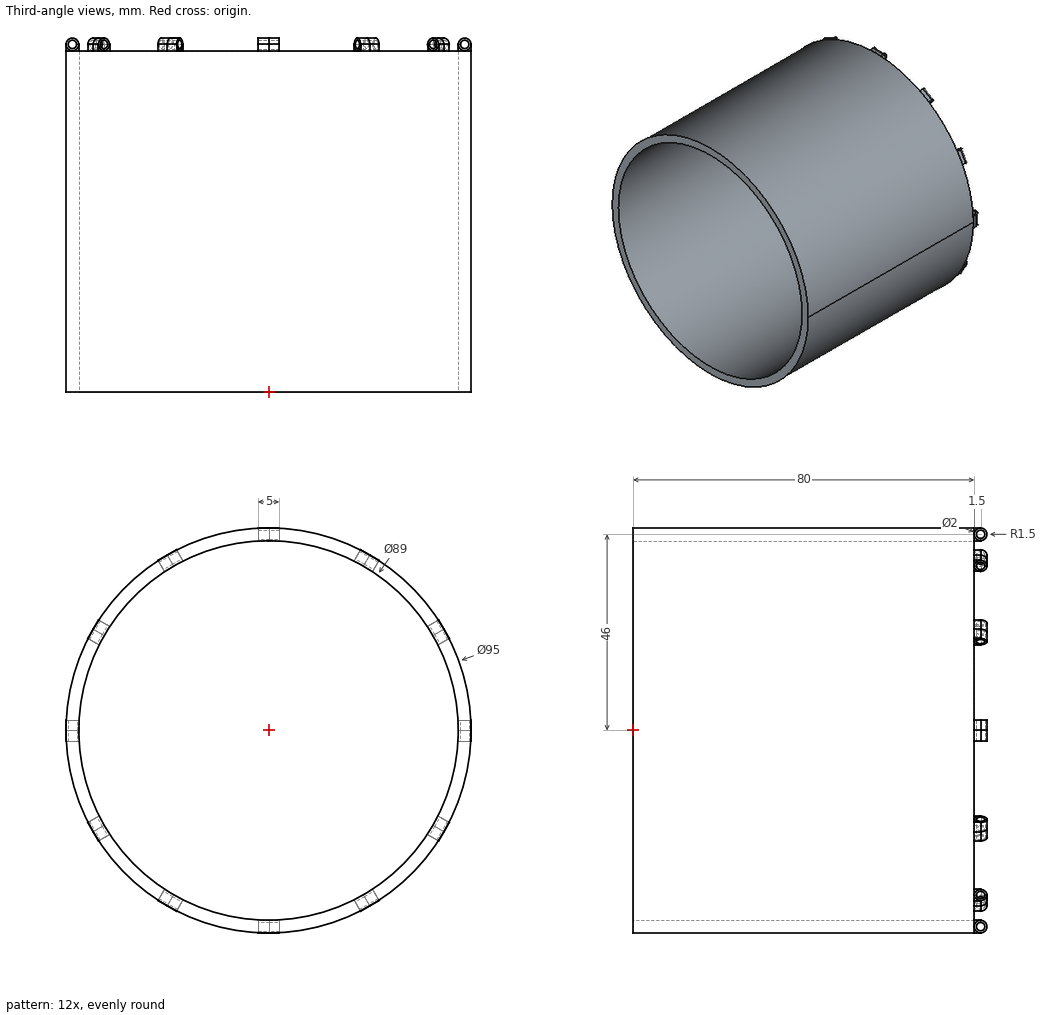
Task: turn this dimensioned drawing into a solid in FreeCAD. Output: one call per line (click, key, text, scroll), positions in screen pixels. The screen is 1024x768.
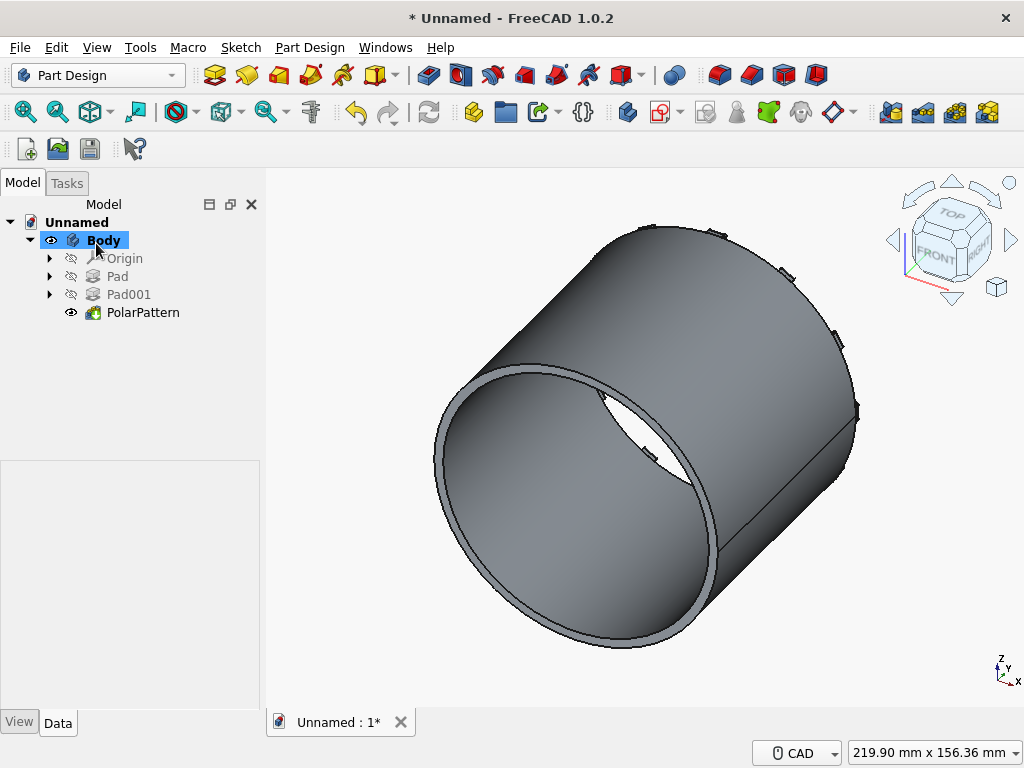
key(0)